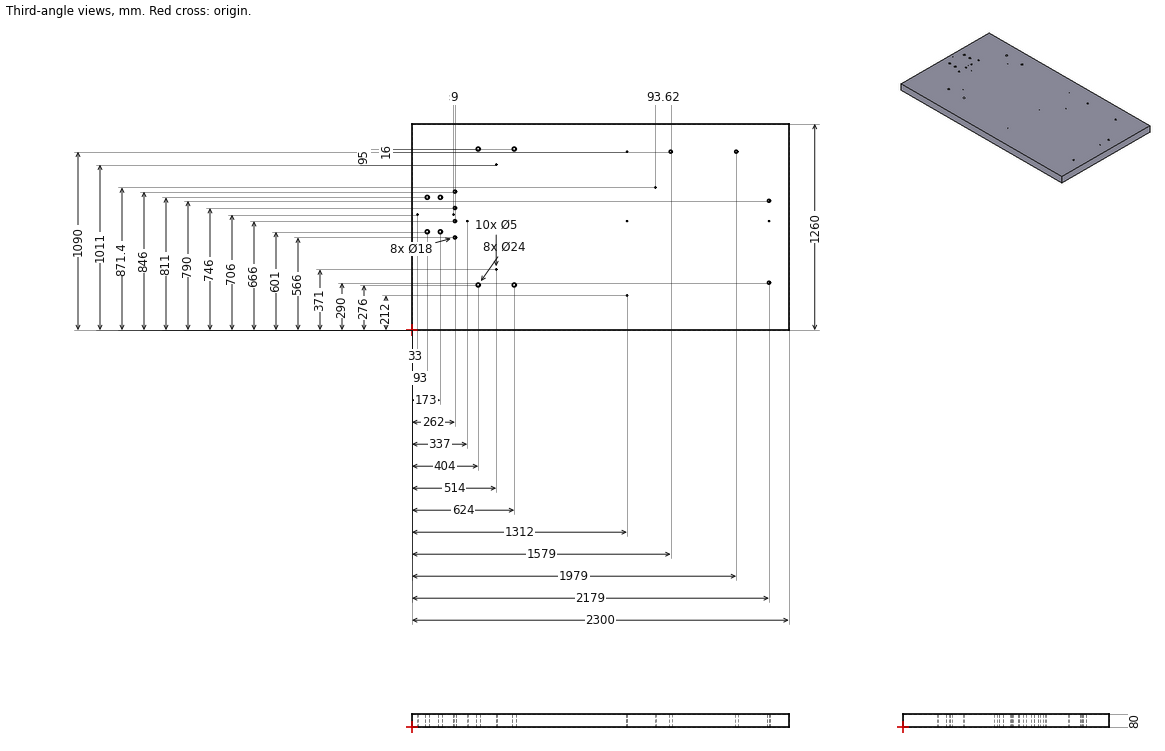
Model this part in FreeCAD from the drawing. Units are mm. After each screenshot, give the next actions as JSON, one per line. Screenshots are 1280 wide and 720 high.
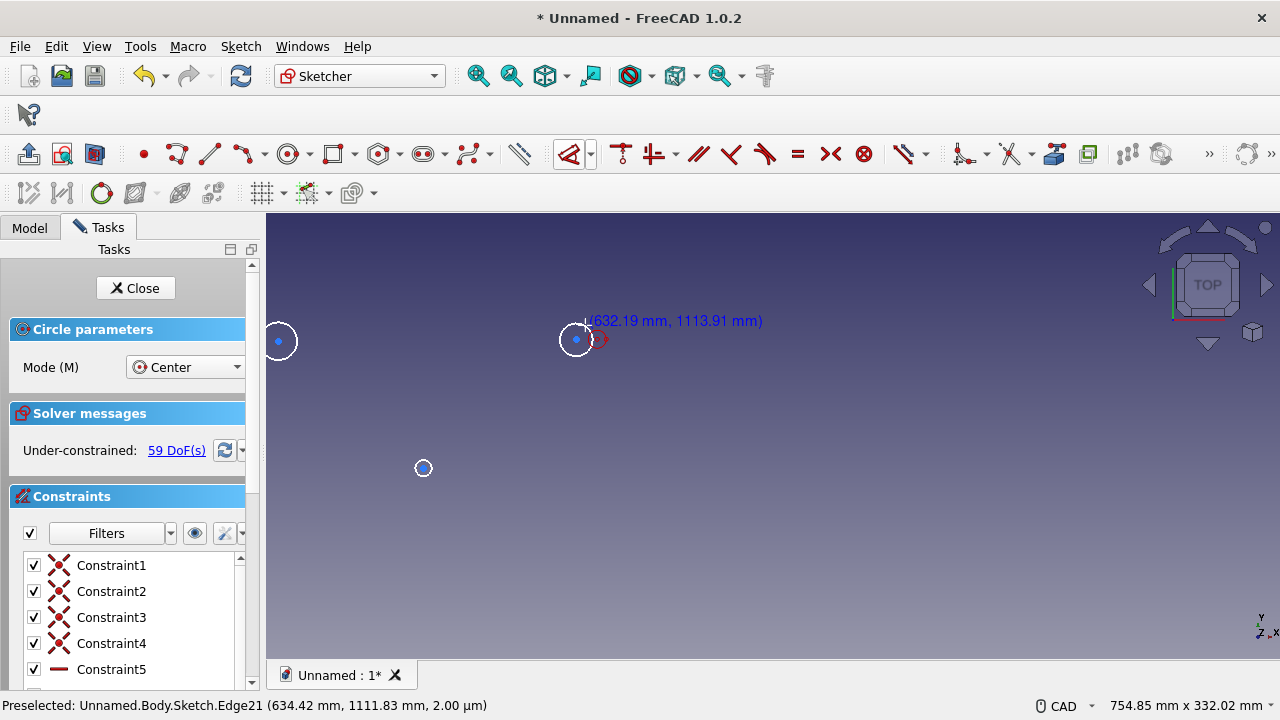
{"action": "scroll", "coordinate": [590, 329], "scroll_direction": "down", "scroll_amount": 9}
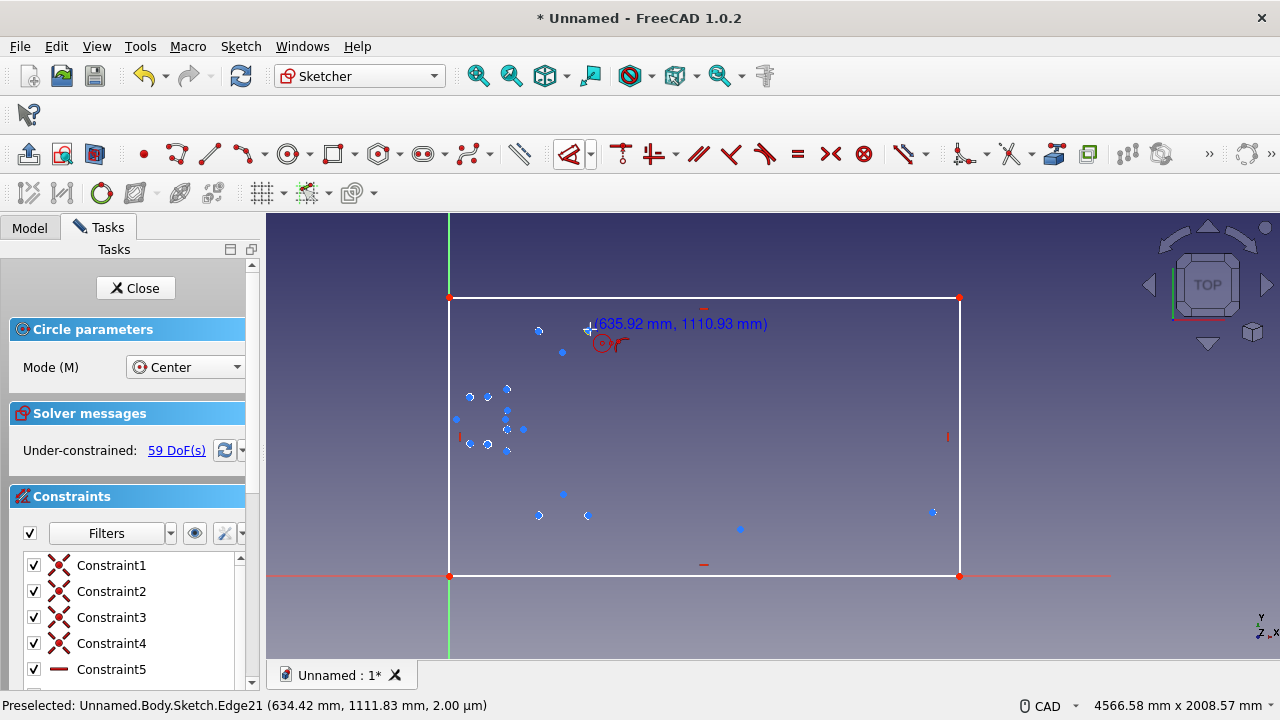
{"action": "scroll", "coordinate": [740, 428], "scroll_direction": "up", "scroll_amount": 19}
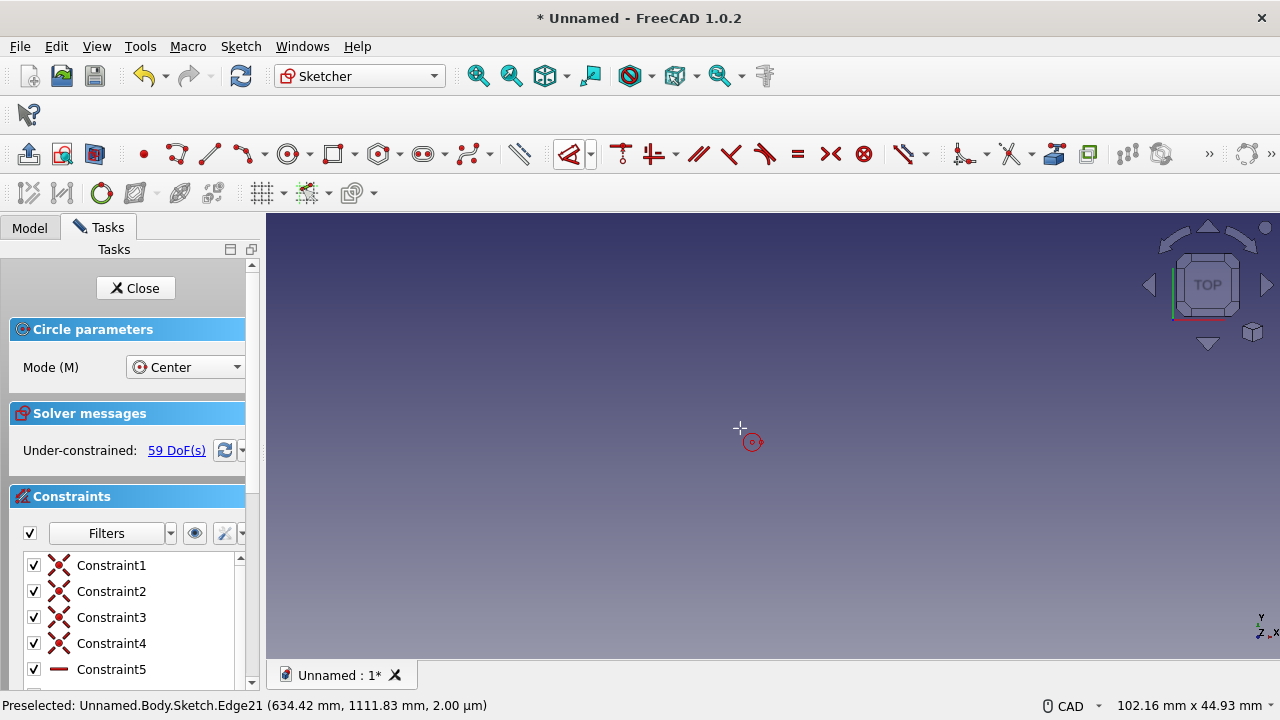
{"action": "scroll", "coordinate": [704, 436], "scroll_direction": "down", "scroll_amount": 15}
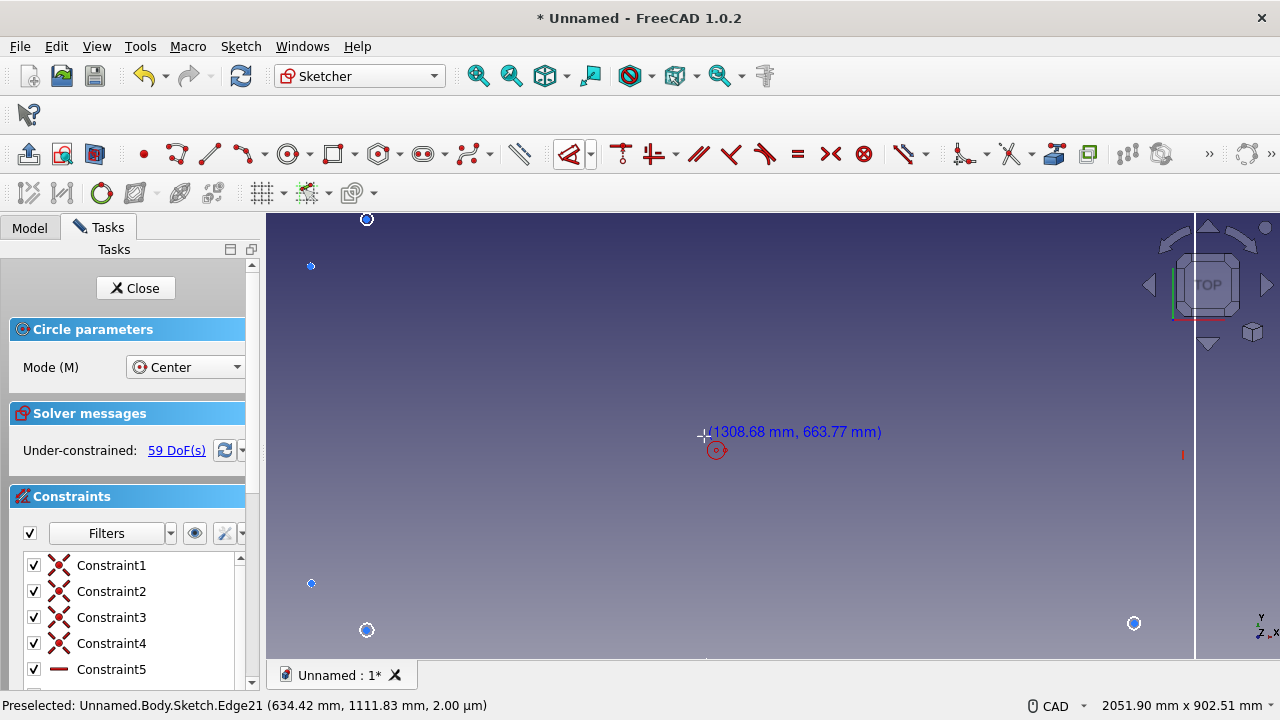
{"action": "scroll", "coordinate": [769, 422], "scroll_direction": "down", "scroll_amount": 4}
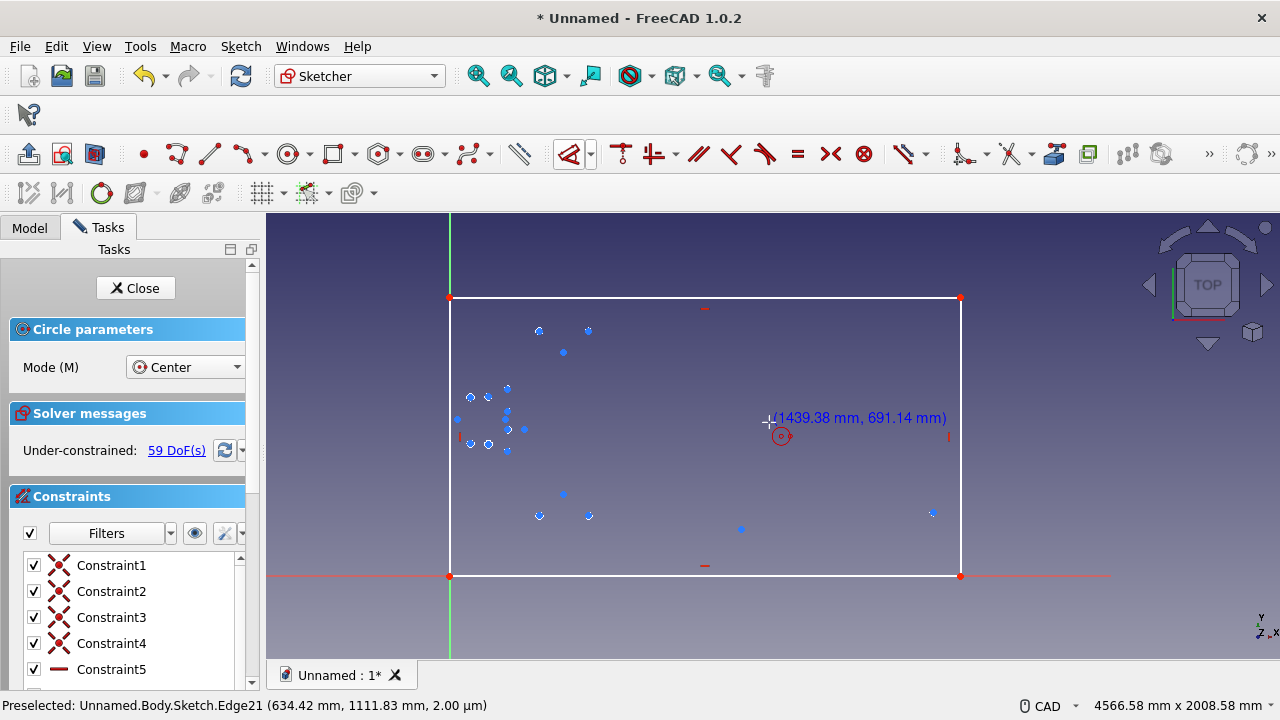
{"action": "left_click", "coordinate": [741, 428]}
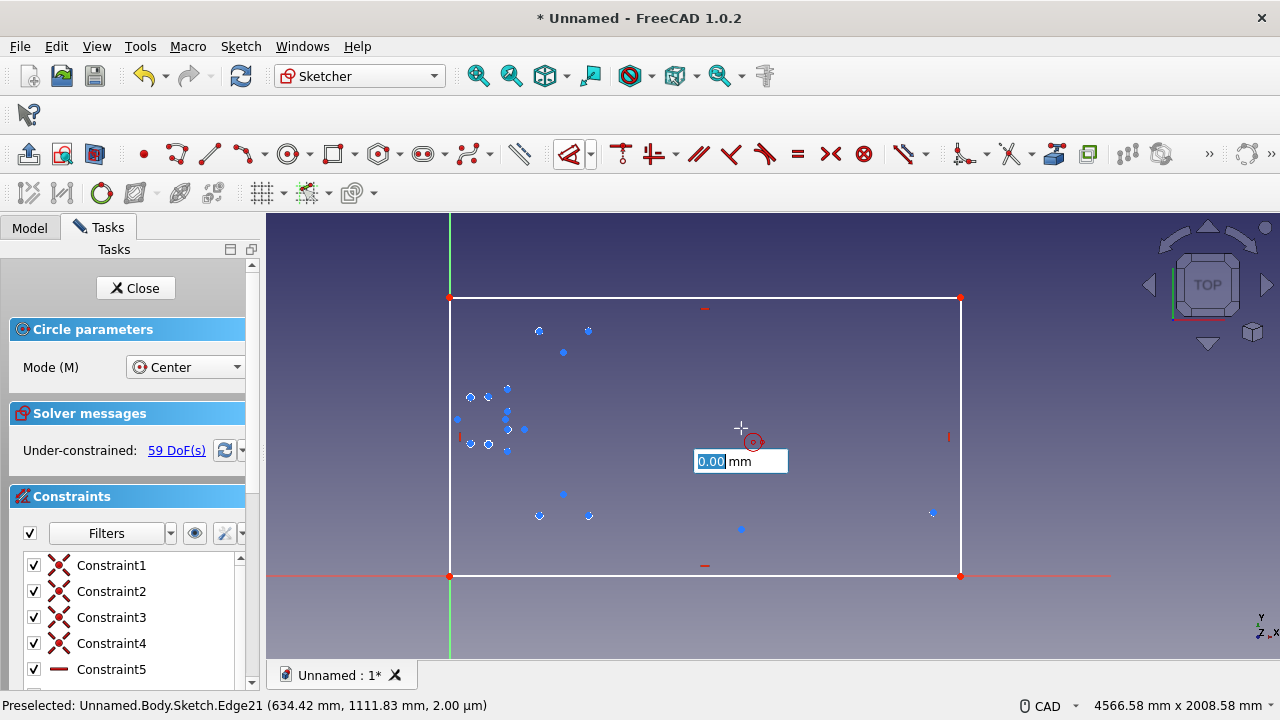
{"action": "scroll", "coordinate": [741, 428], "scroll_direction": "up", "scroll_amount": 17}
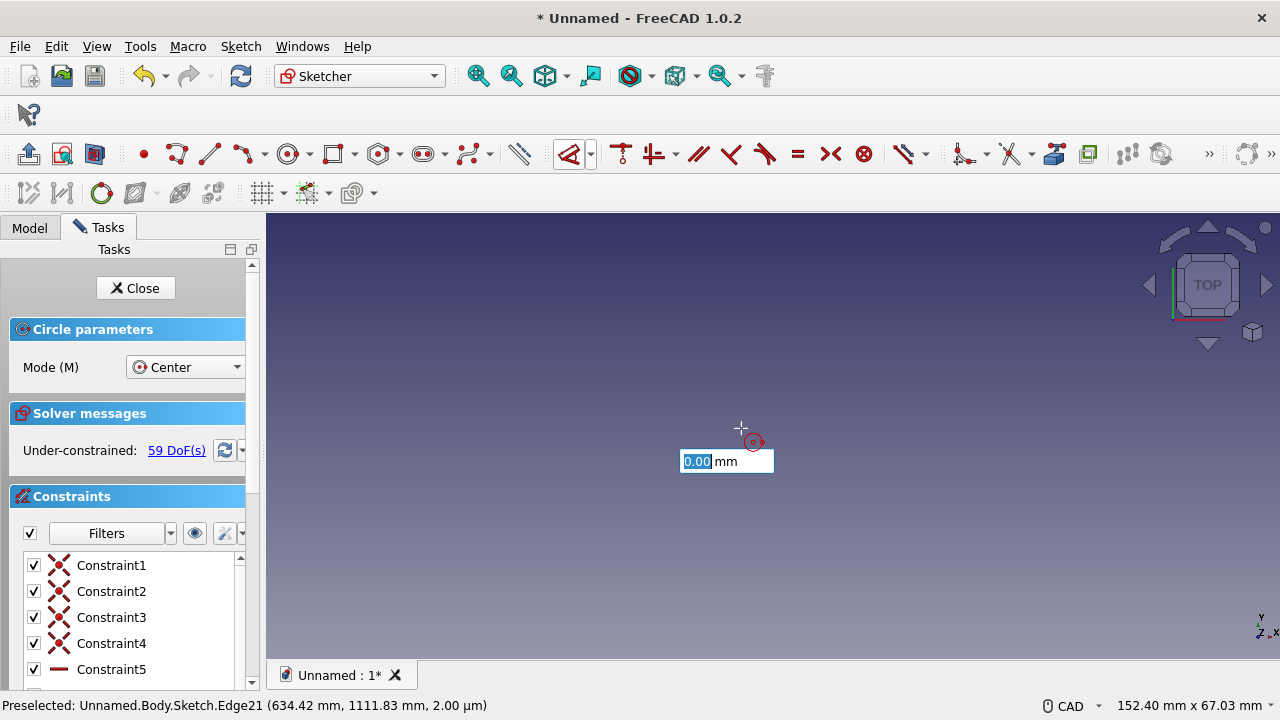
{"action": "left_click", "coordinate": [739, 411]}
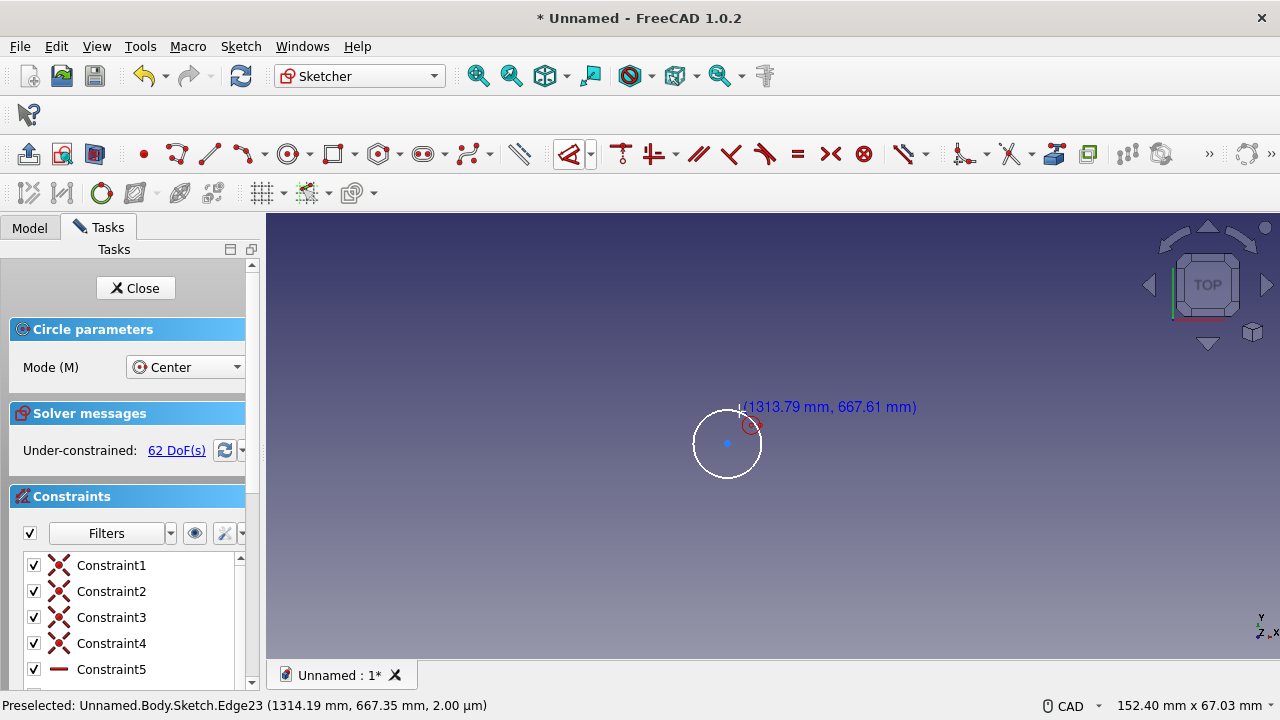
{"action": "scroll", "coordinate": [741, 428], "scroll_direction": "down", "scroll_amount": 17}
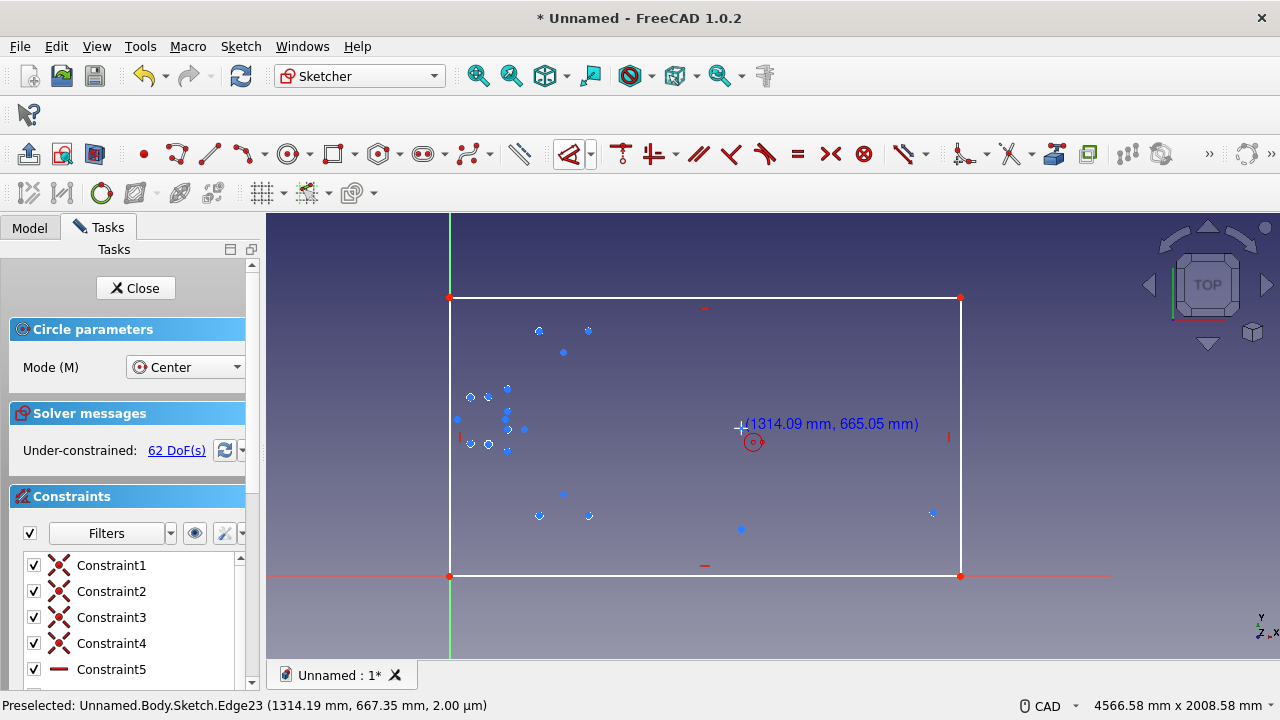
{"action": "scroll", "coordinate": [779, 383], "scroll_direction": "up", "scroll_amount": 19}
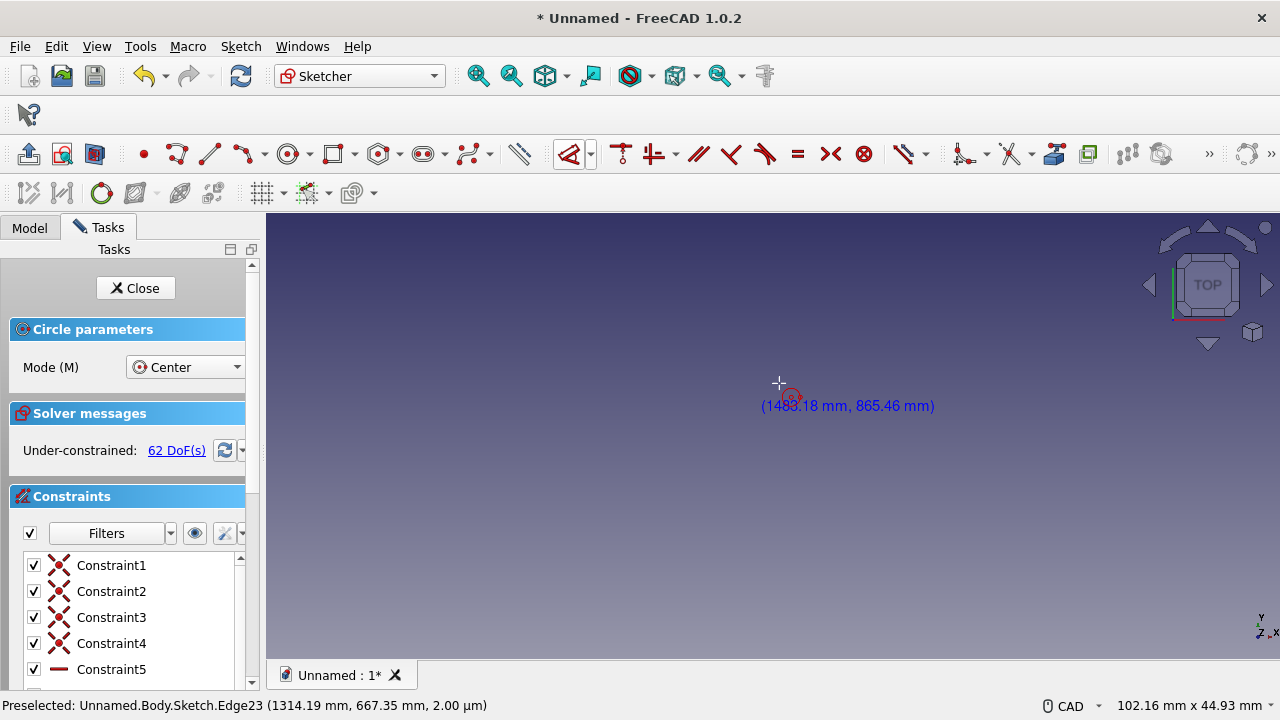
{"action": "scroll", "coordinate": [704, 436], "scroll_direction": "down", "scroll_amount": 15}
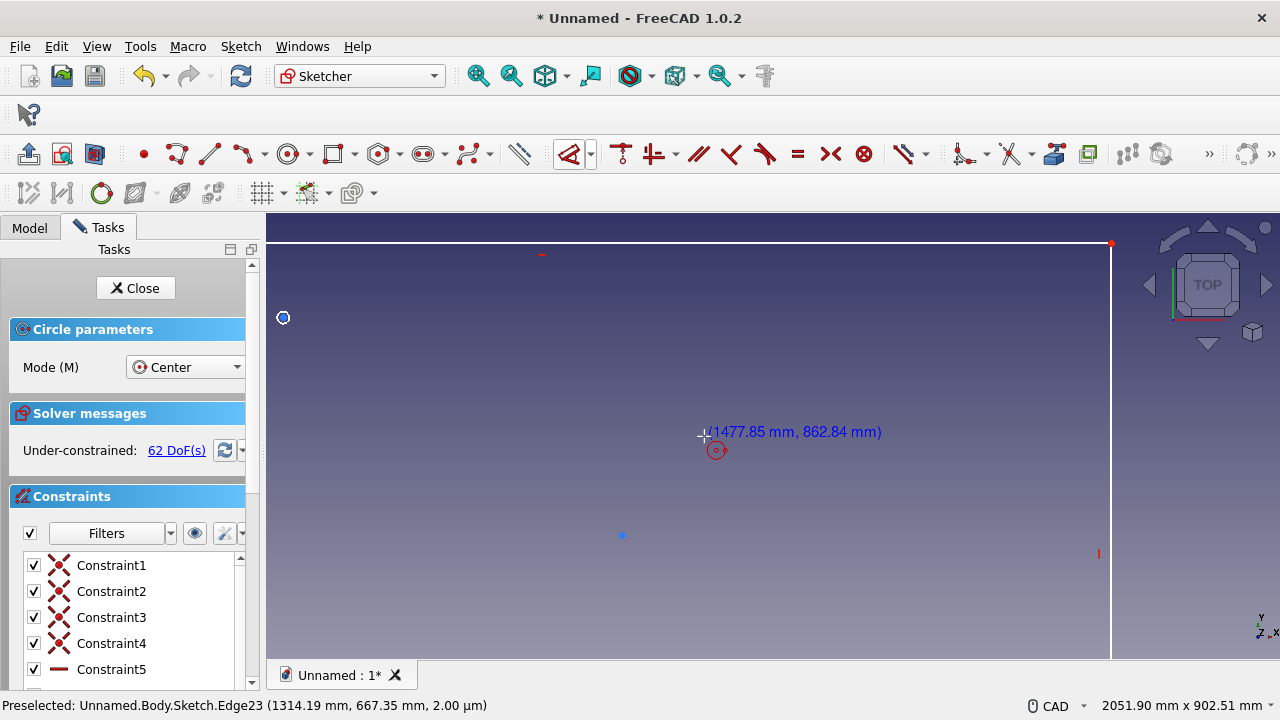
{"action": "scroll", "coordinate": [837, 342], "scroll_direction": "down", "scroll_amount": 4}